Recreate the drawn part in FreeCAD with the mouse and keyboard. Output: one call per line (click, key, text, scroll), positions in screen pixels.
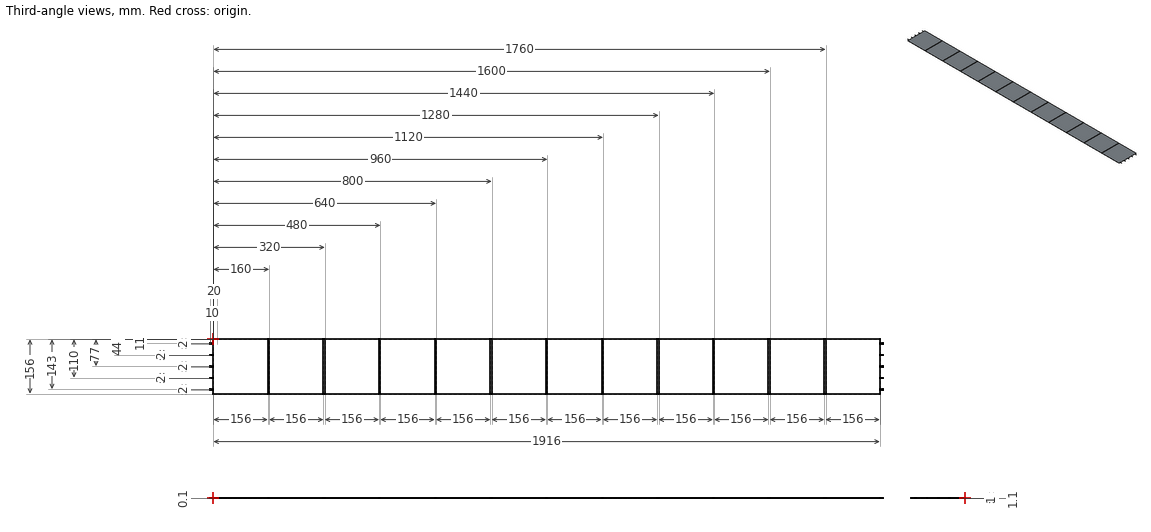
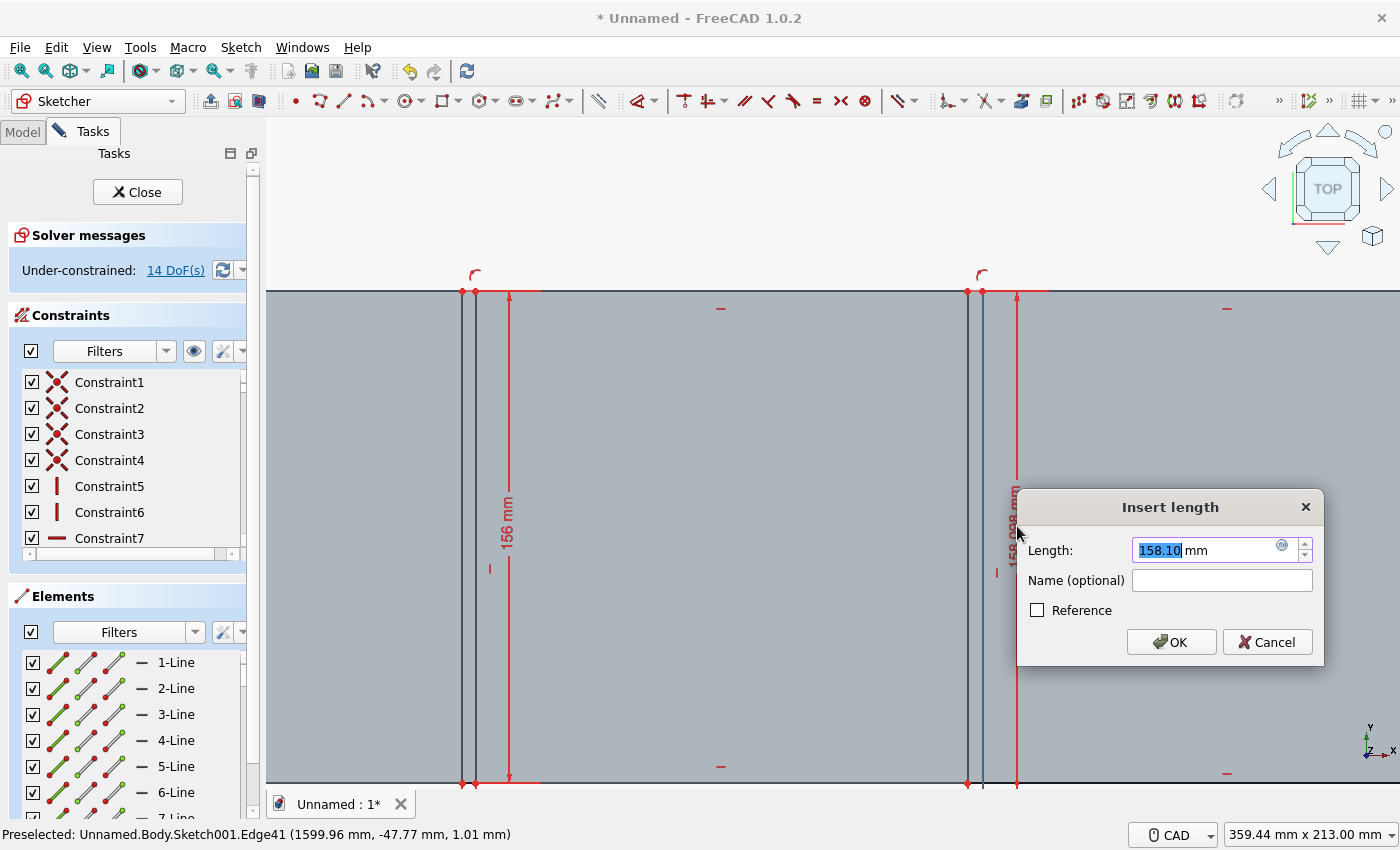
text(156)
key(Return)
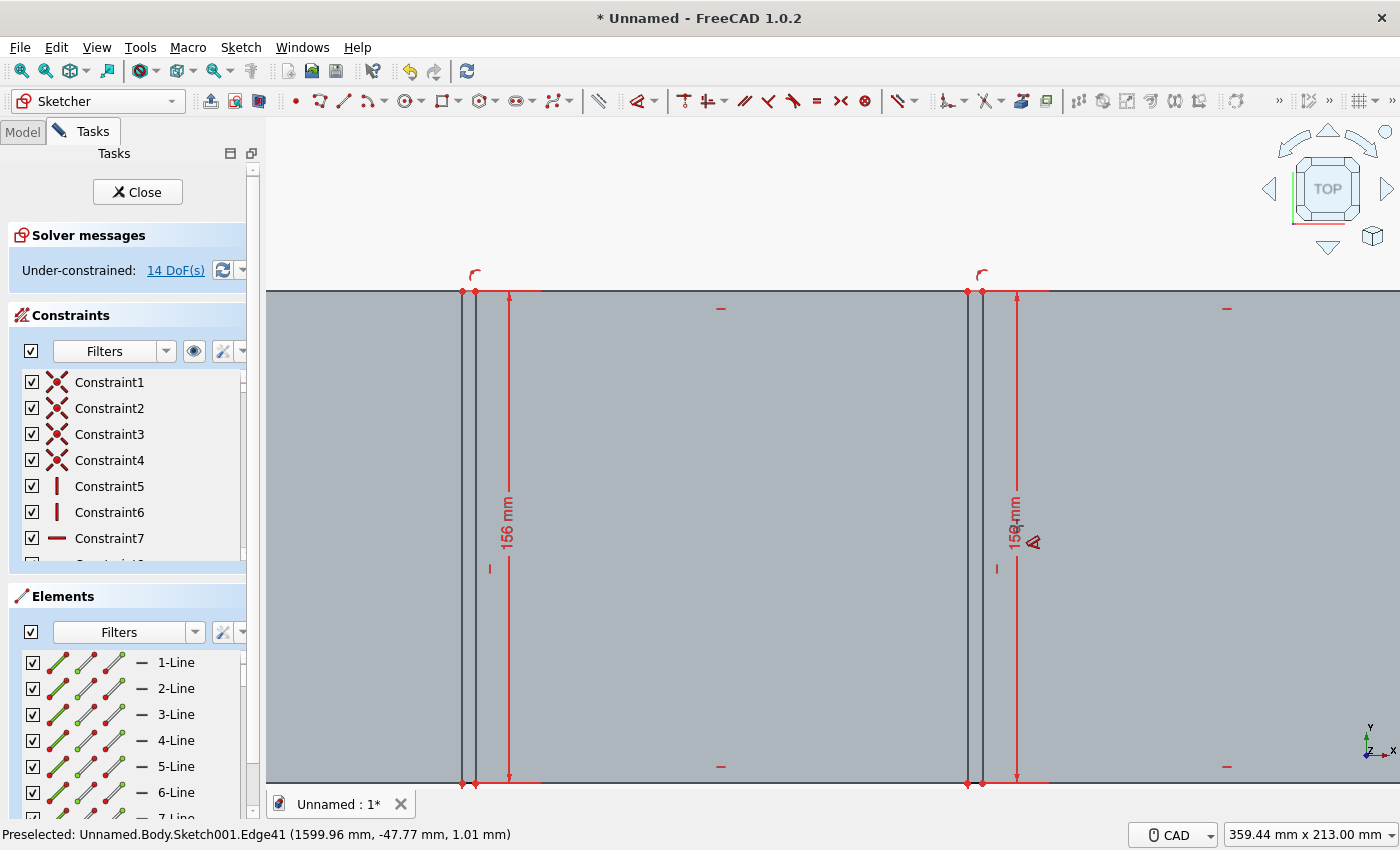
scroll(990, 442, down, 11)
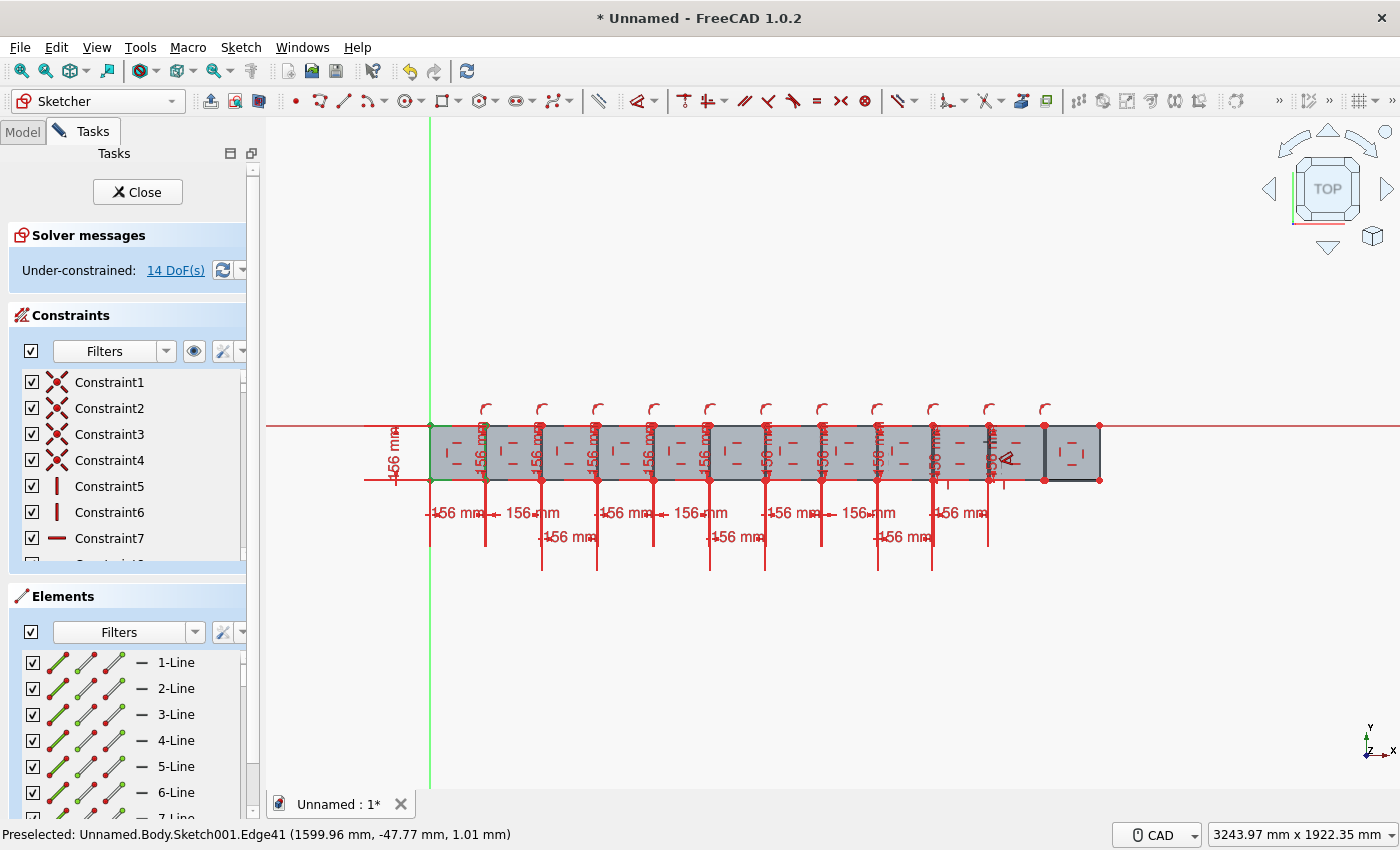
click(1006, 480)
click(1036, 514)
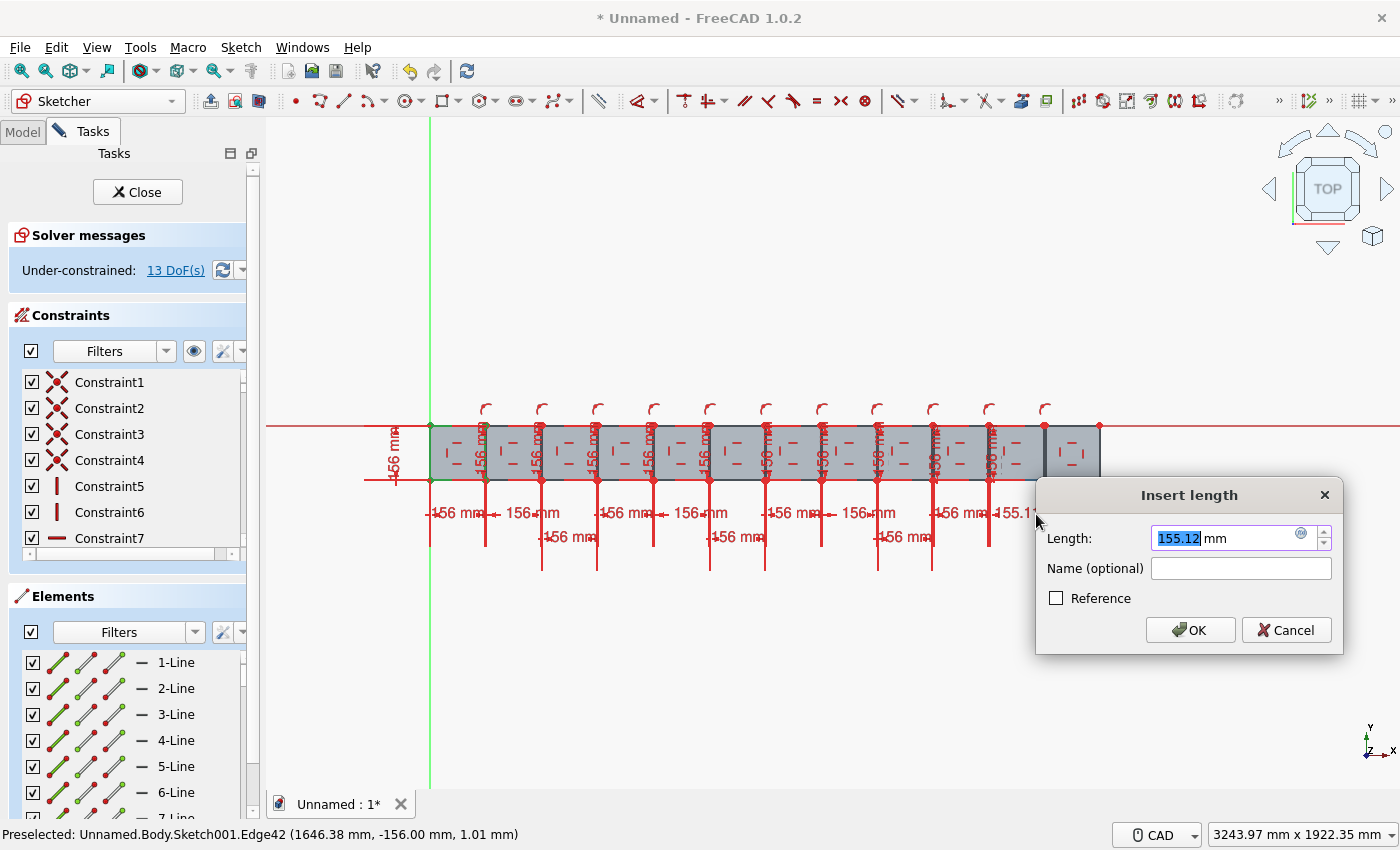
text(156)
key(Return)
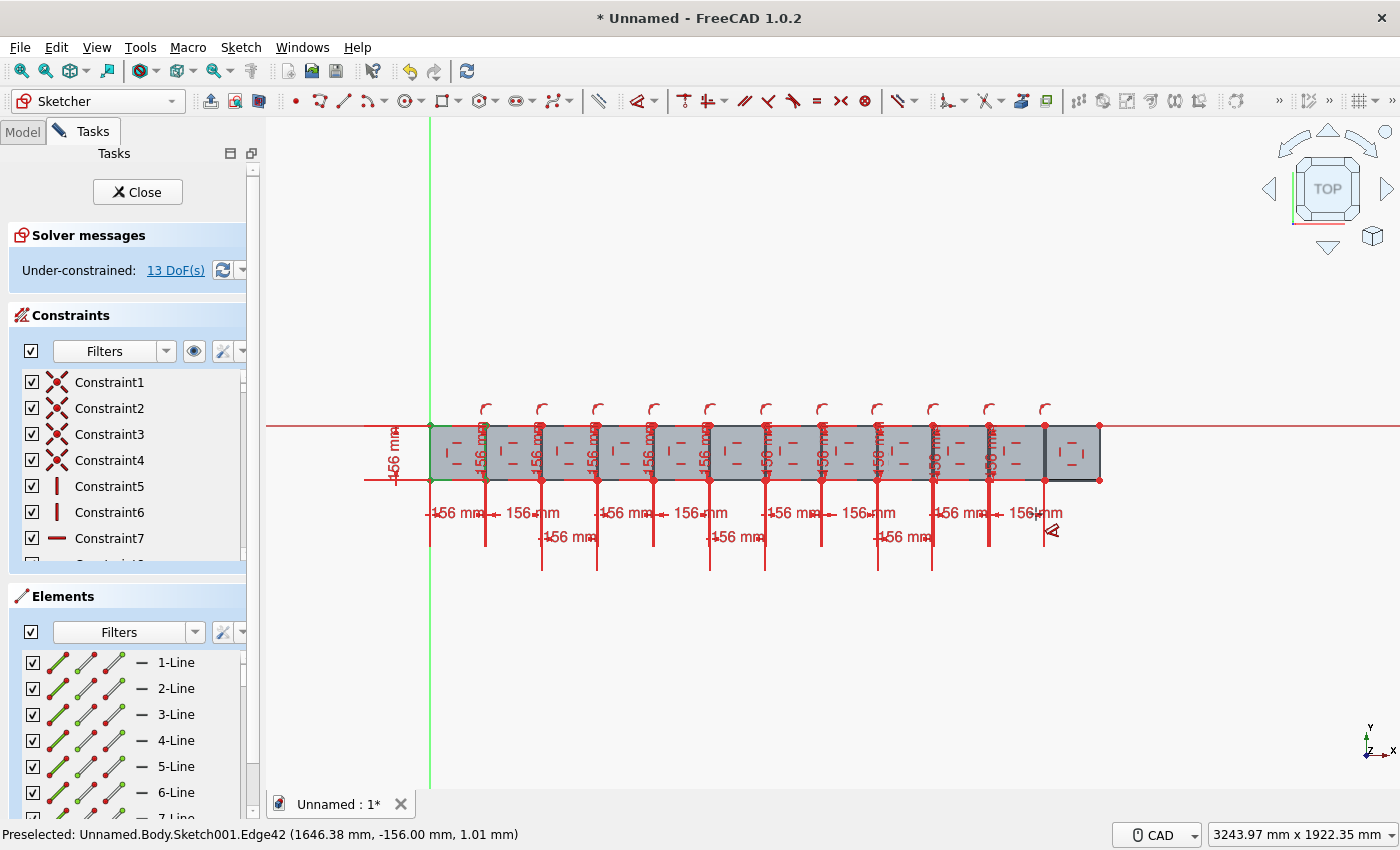
scroll(1046, 442, up, 11)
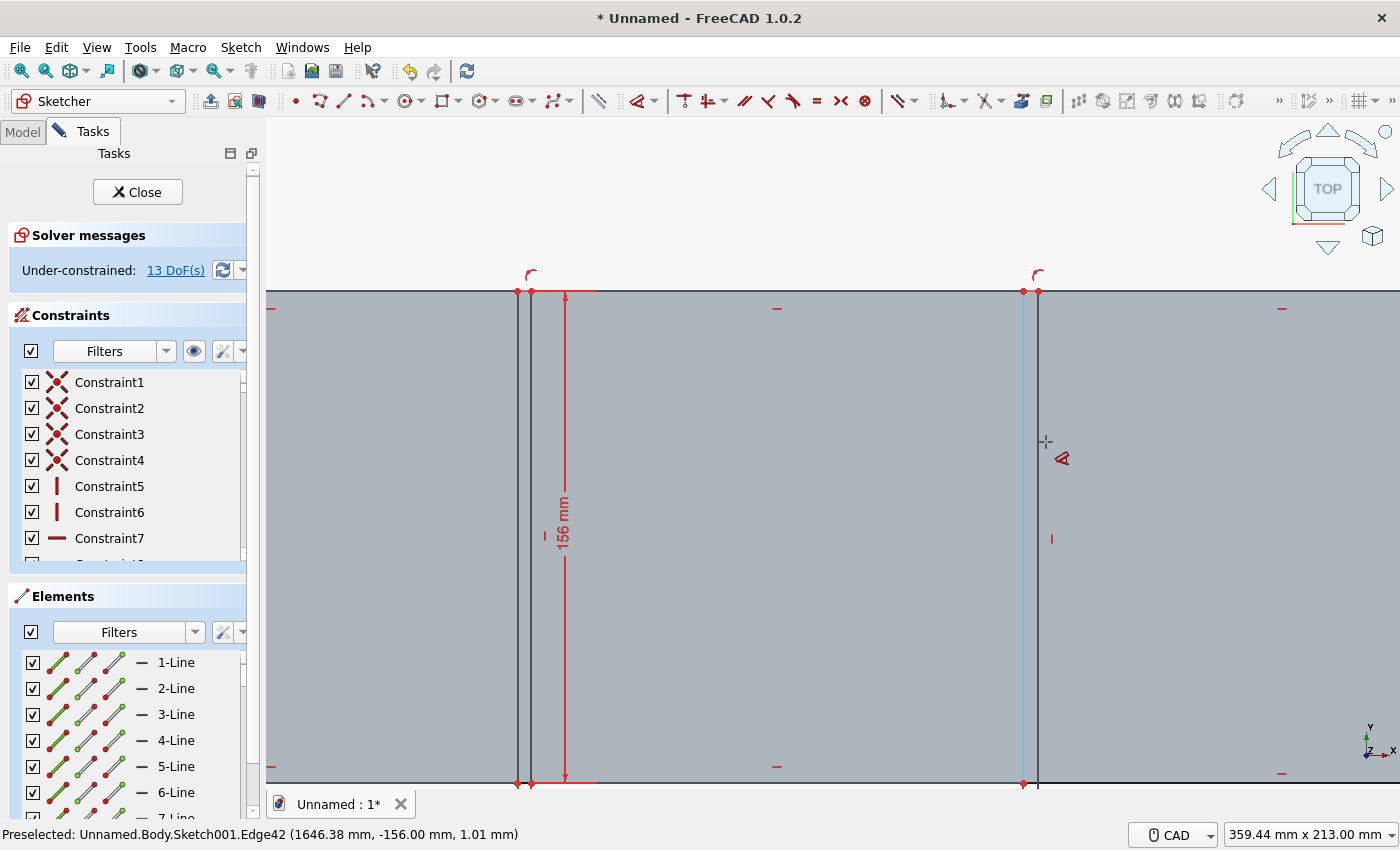
click(1038, 441)
click(1072, 526)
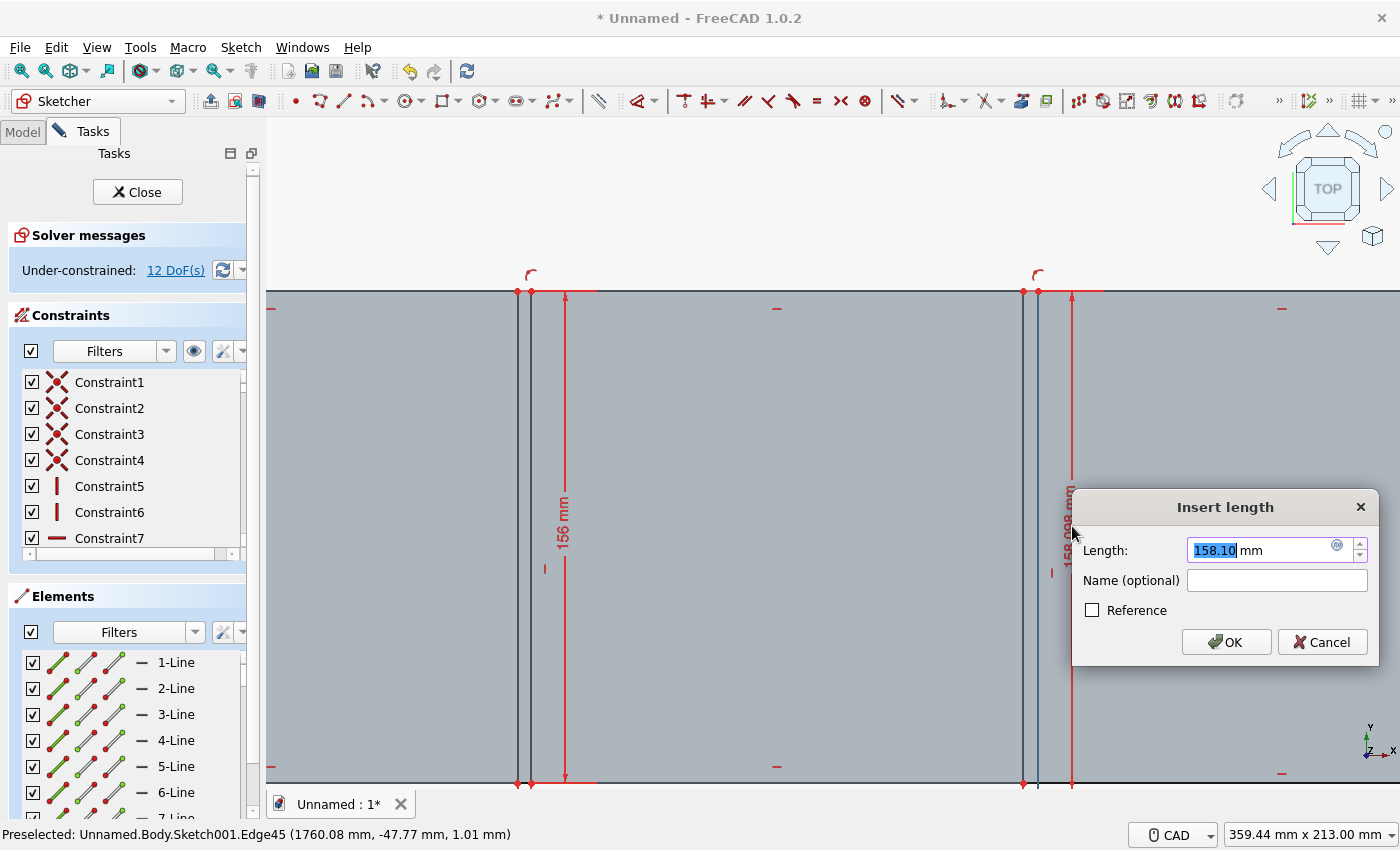
text(156)
key(Return)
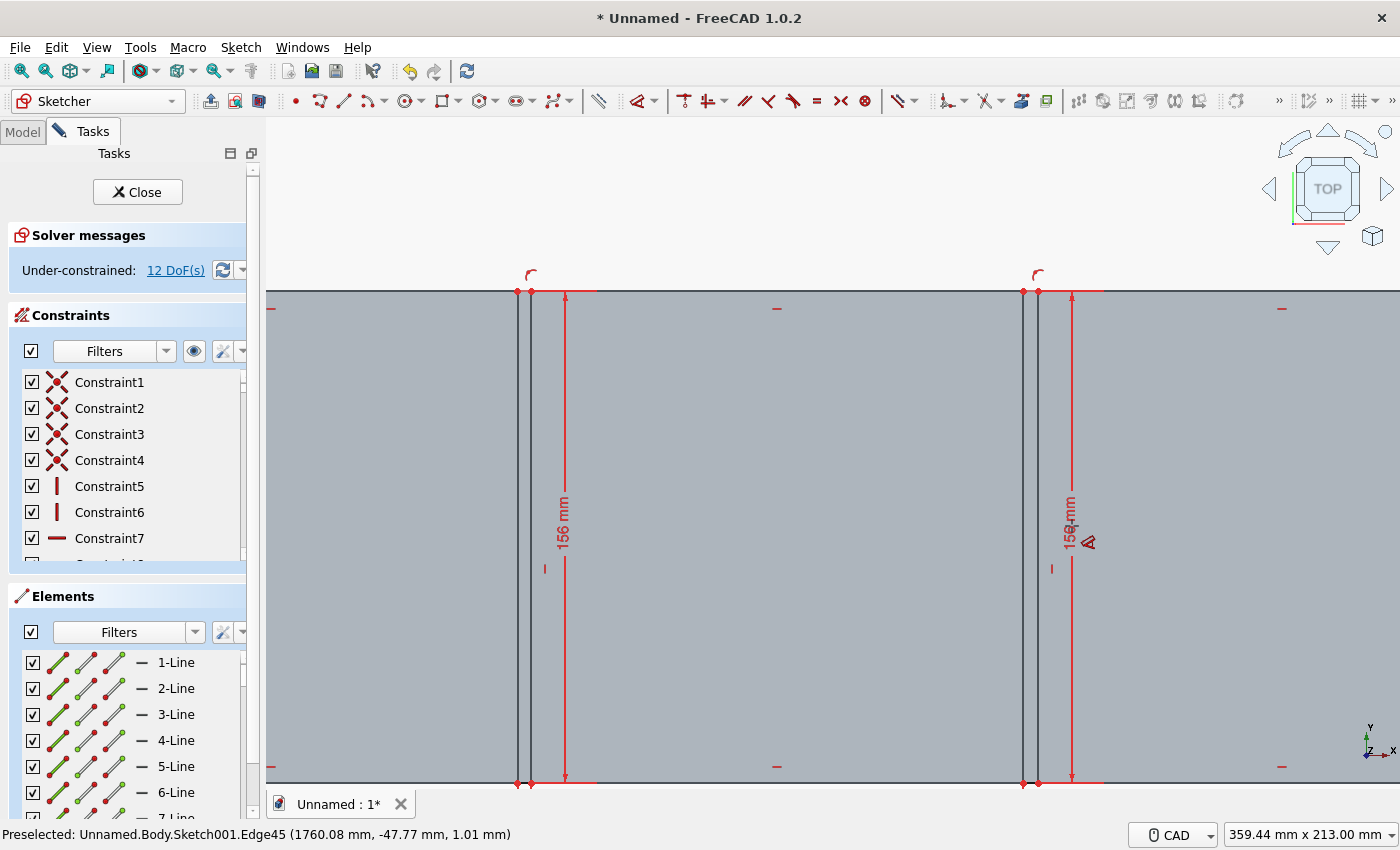
scroll(1046, 442, down, 11)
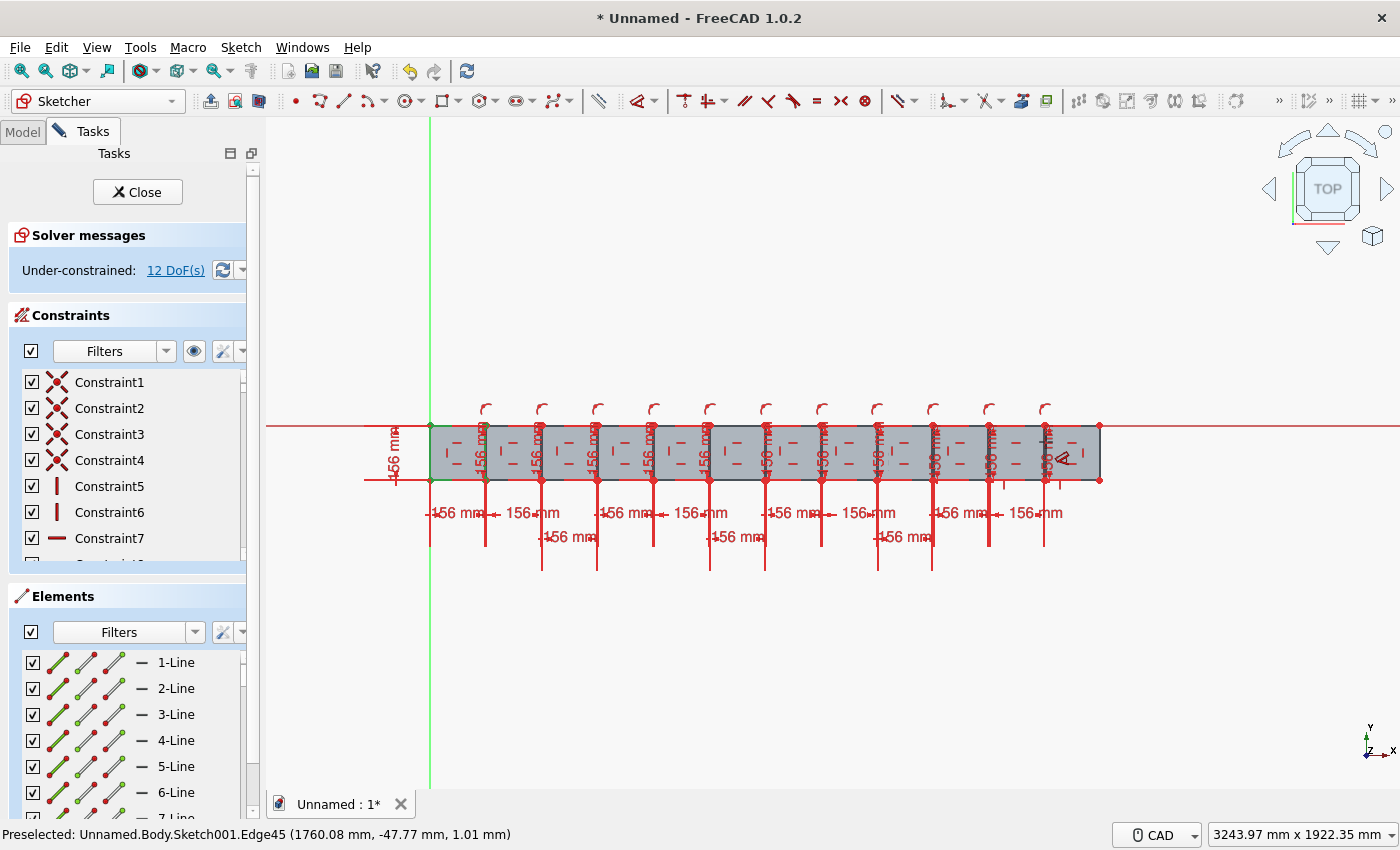
click(1062, 480)
click(1073, 538)